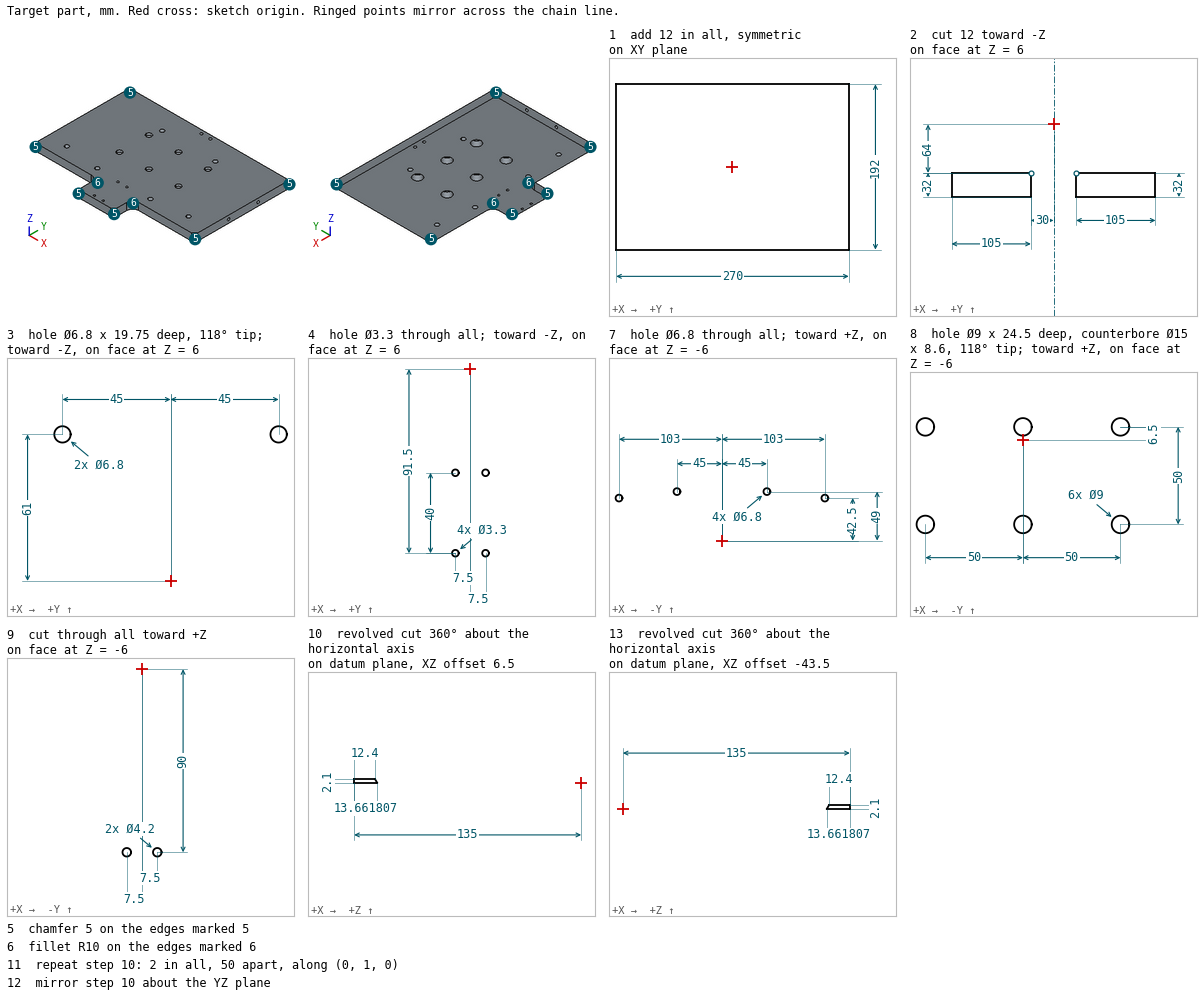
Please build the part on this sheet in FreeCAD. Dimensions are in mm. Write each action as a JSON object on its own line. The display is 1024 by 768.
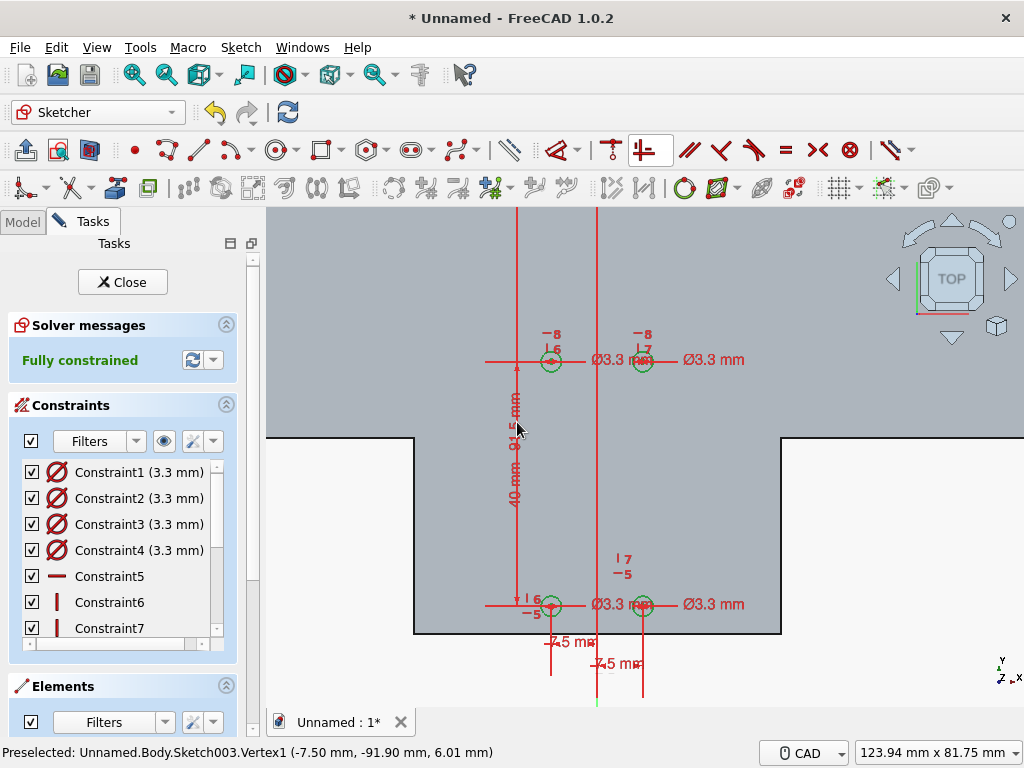
{"action": "left_click", "coordinate": [123, 282]}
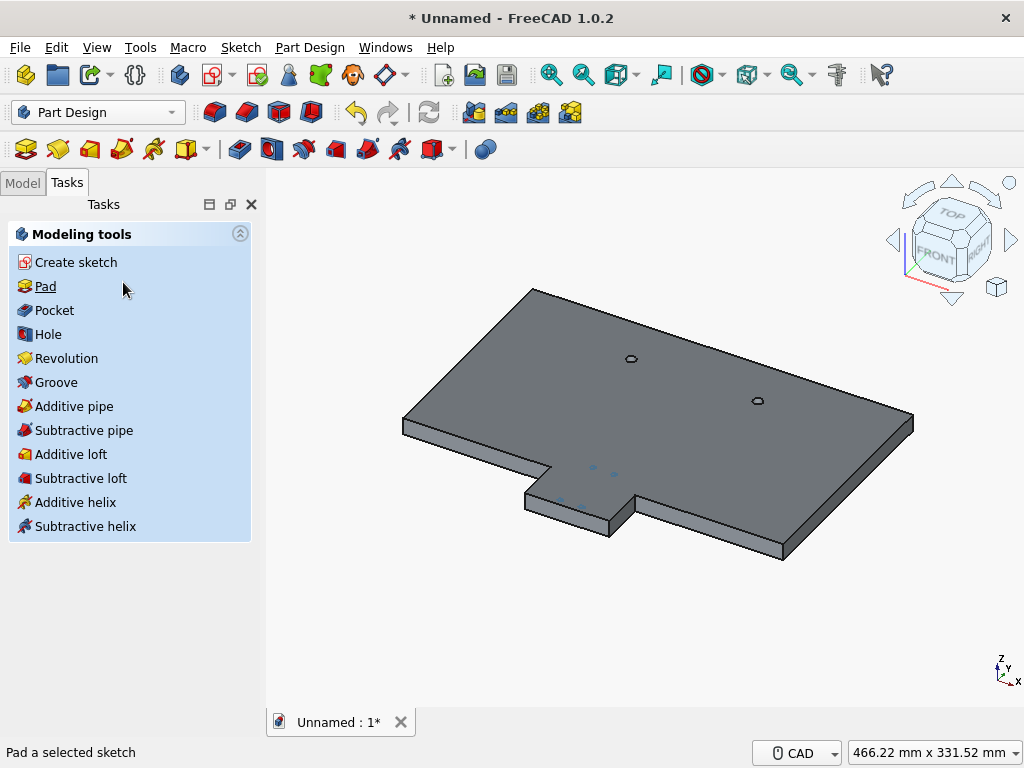
{"action": "left_click", "coordinate": [272, 150]}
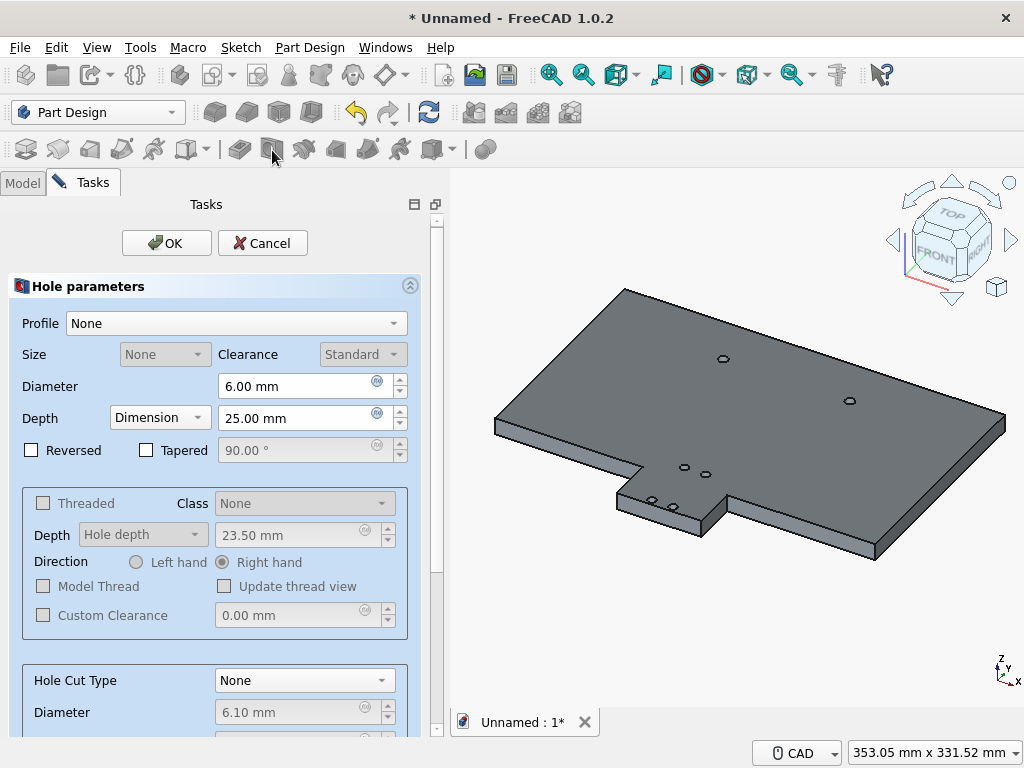
{"action": "triple_click", "coordinate": [305, 386]}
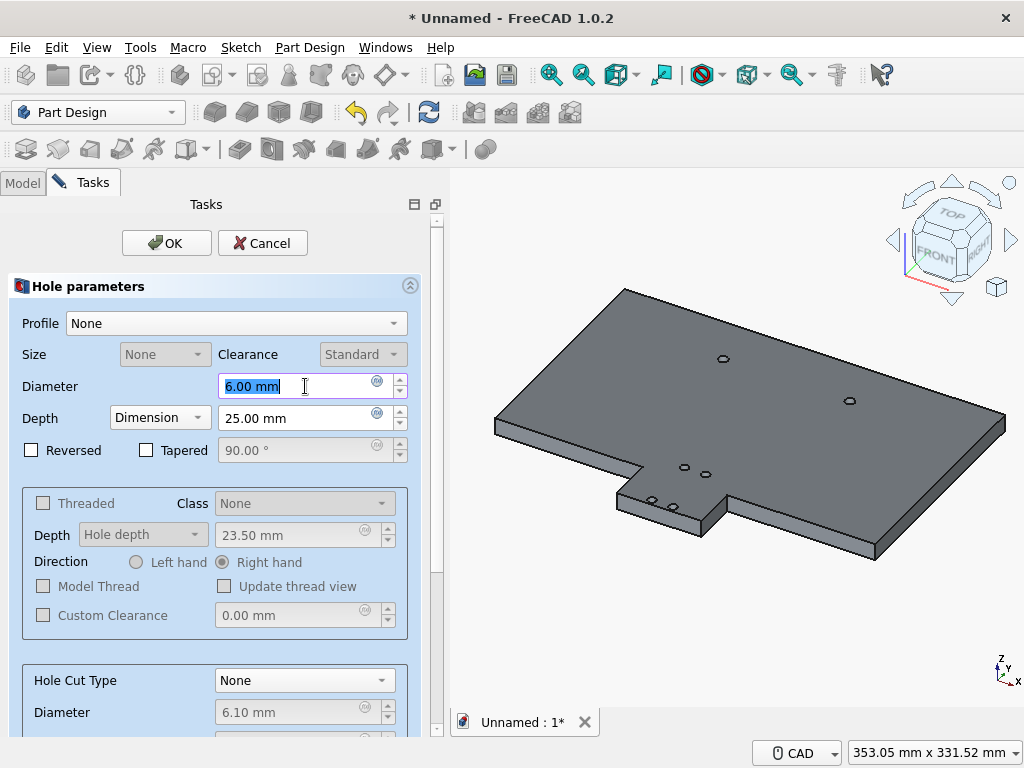
{"action": "type", "text": "3.3"}
{"action": "key", "text": "Tab"}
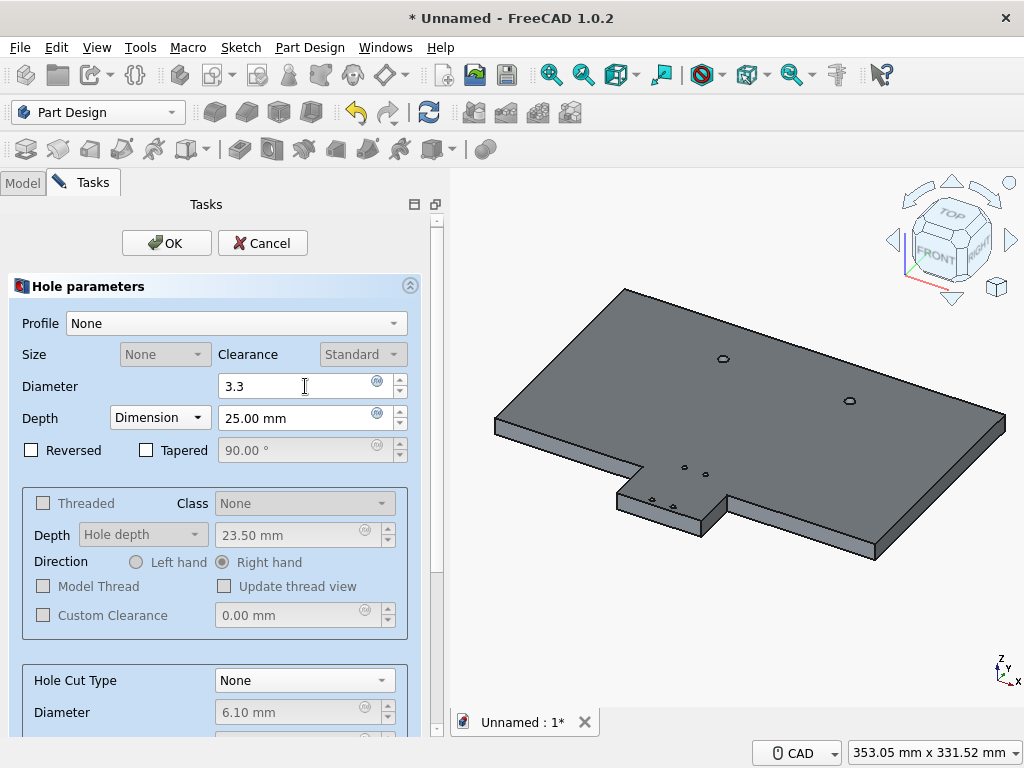
{"action": "left_click", "coordinate": [161, 418]}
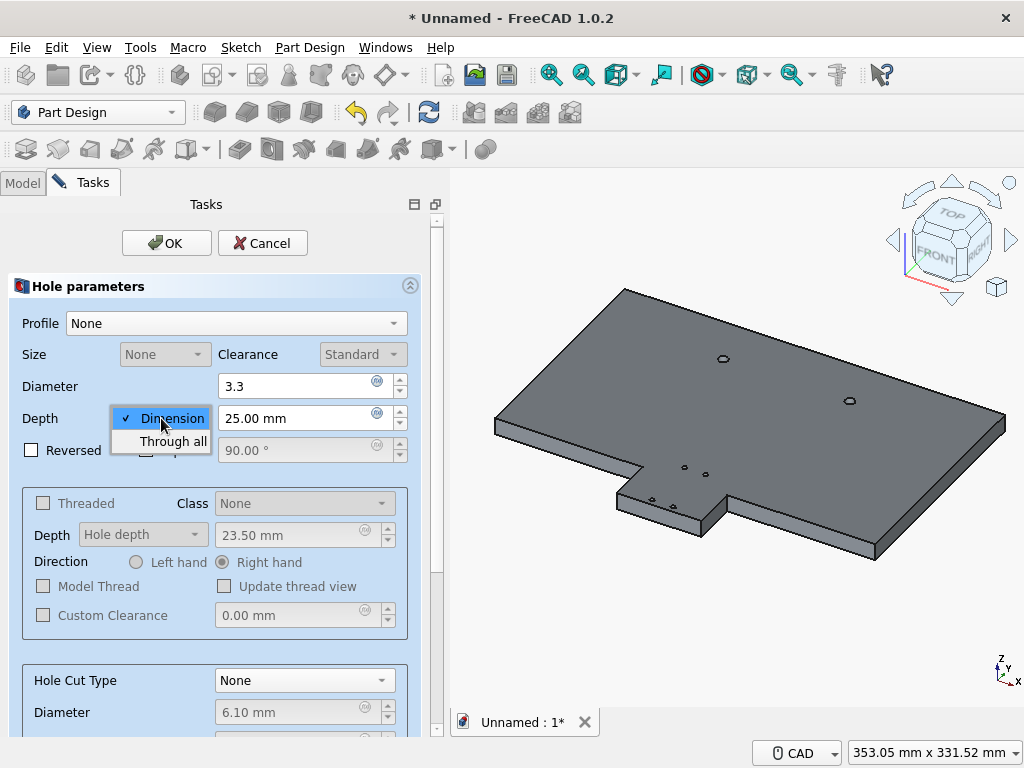
{"action": "left_click", "coordinate": [160, 442]}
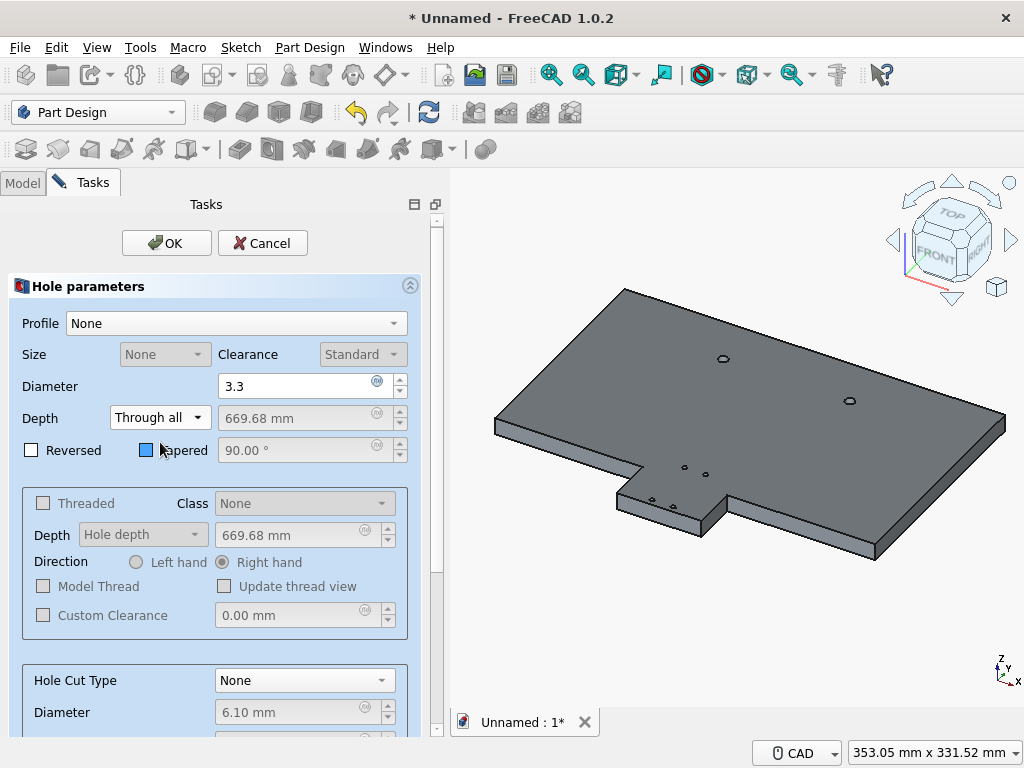
{"action": "left_click", "coordinate": [167, 243]}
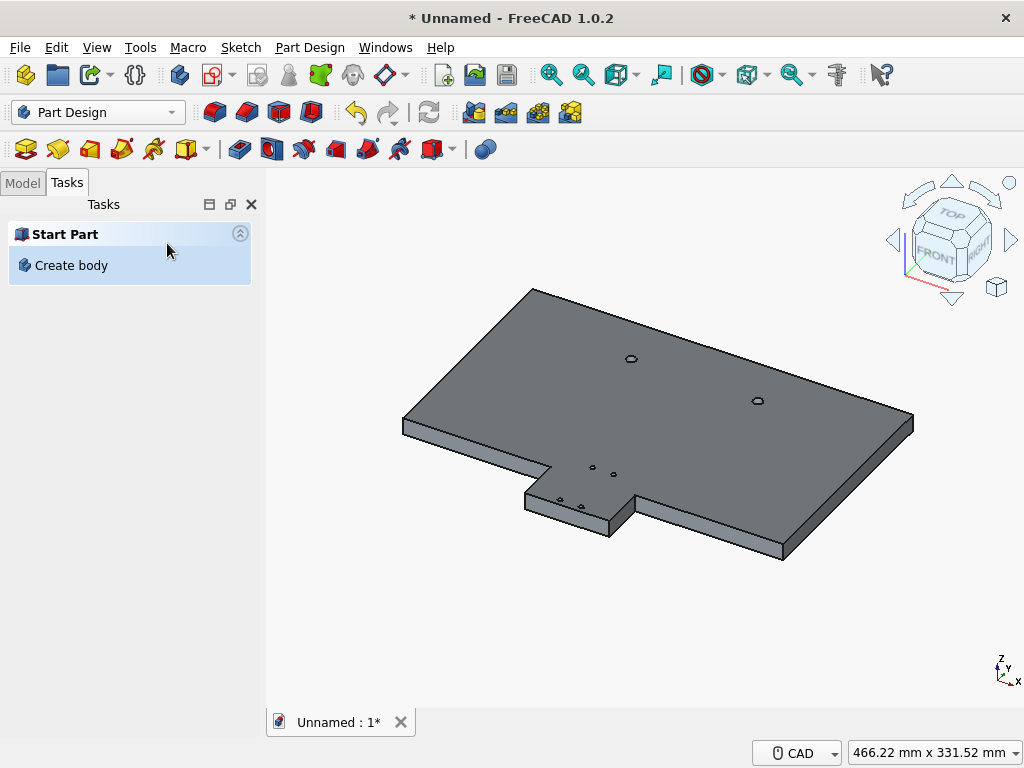
{"action": "left_click", "coordinate": [609, 528]}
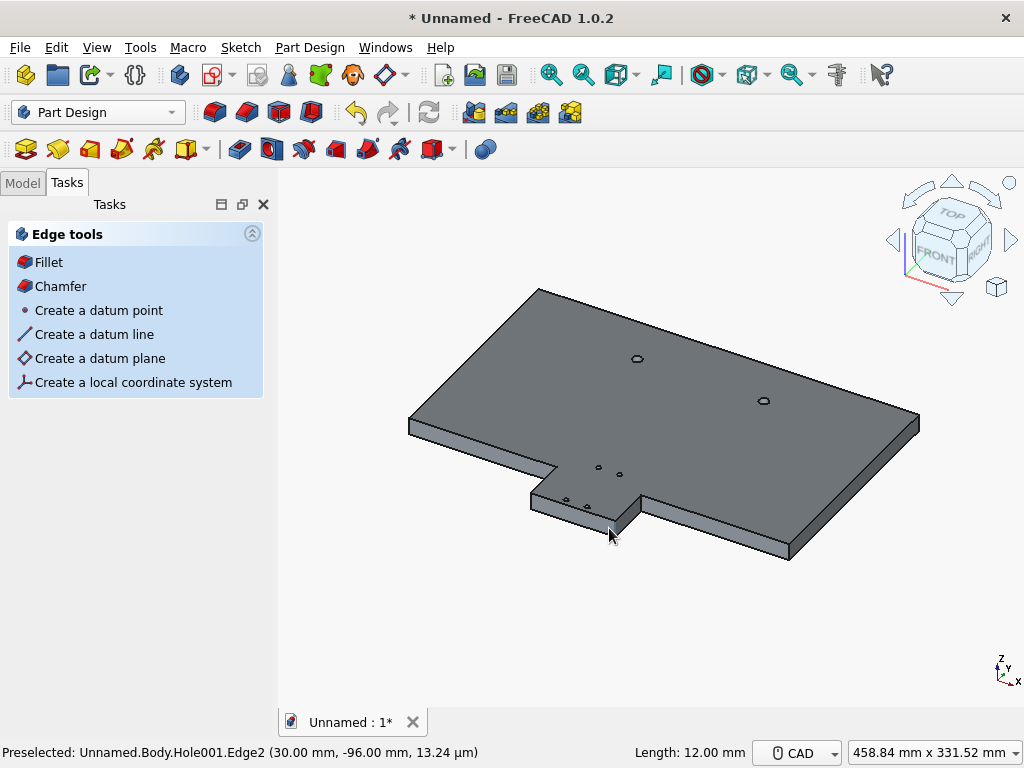
{"action": "left_click", "coordinate": [789, 551], "text": "ctrl"}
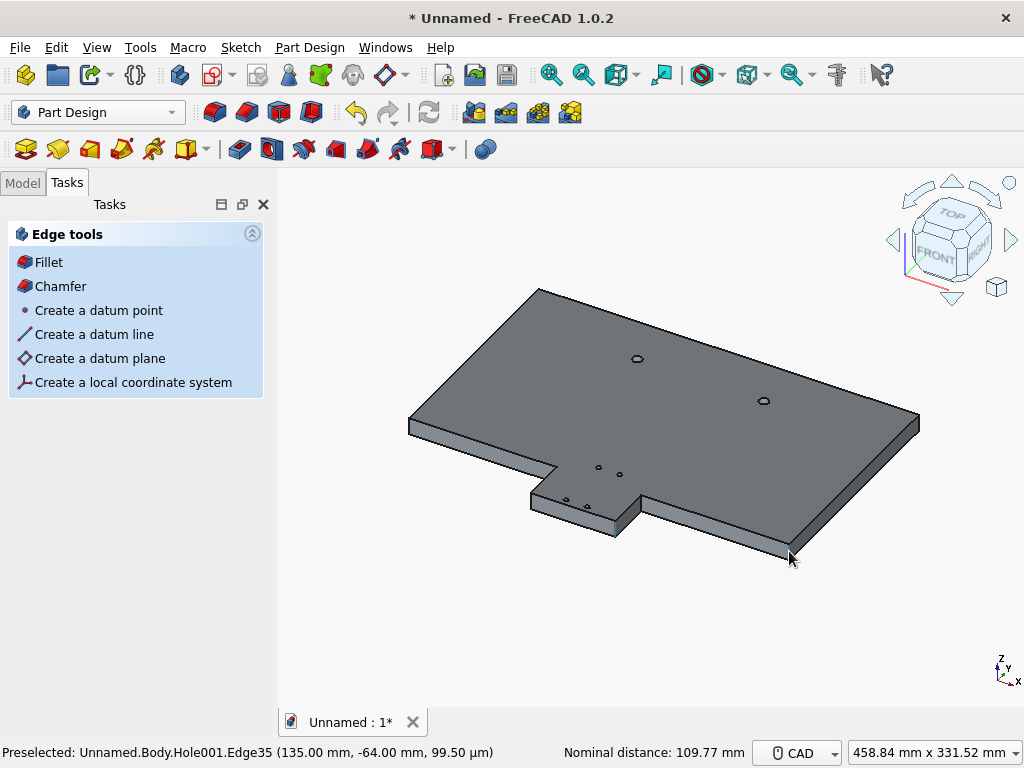
{"action": "scroll", "coordinate": [409, 425], "scroll_direction": "up", "scroll_amount": 4}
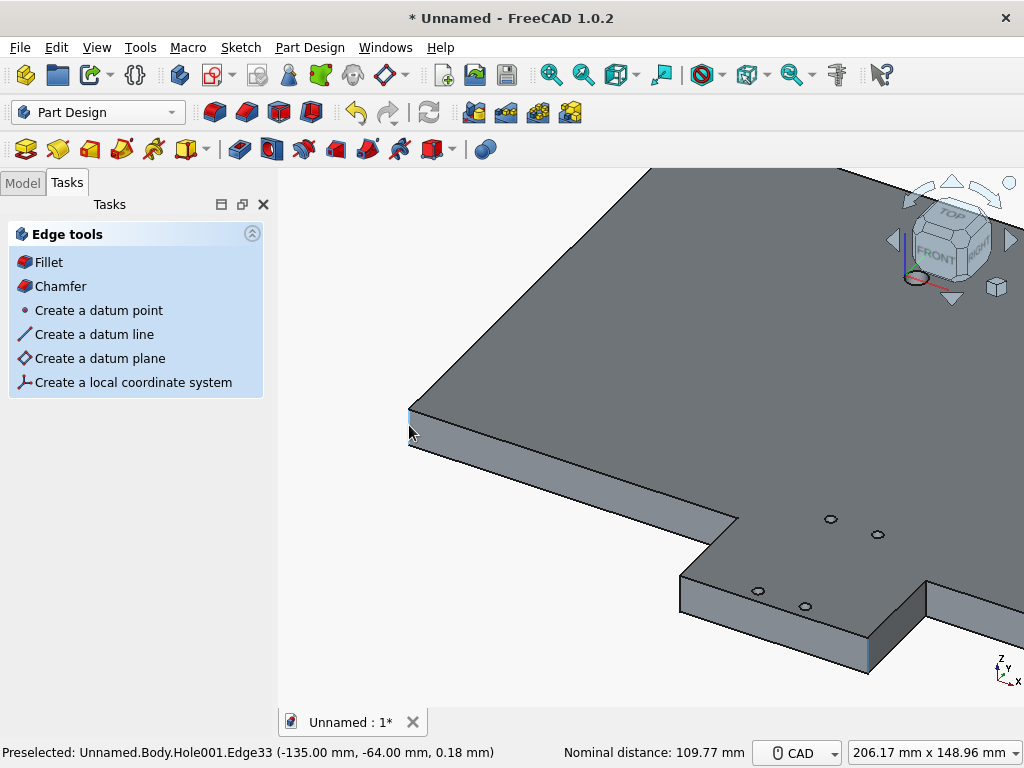
{"action": "key", "text": "v f"}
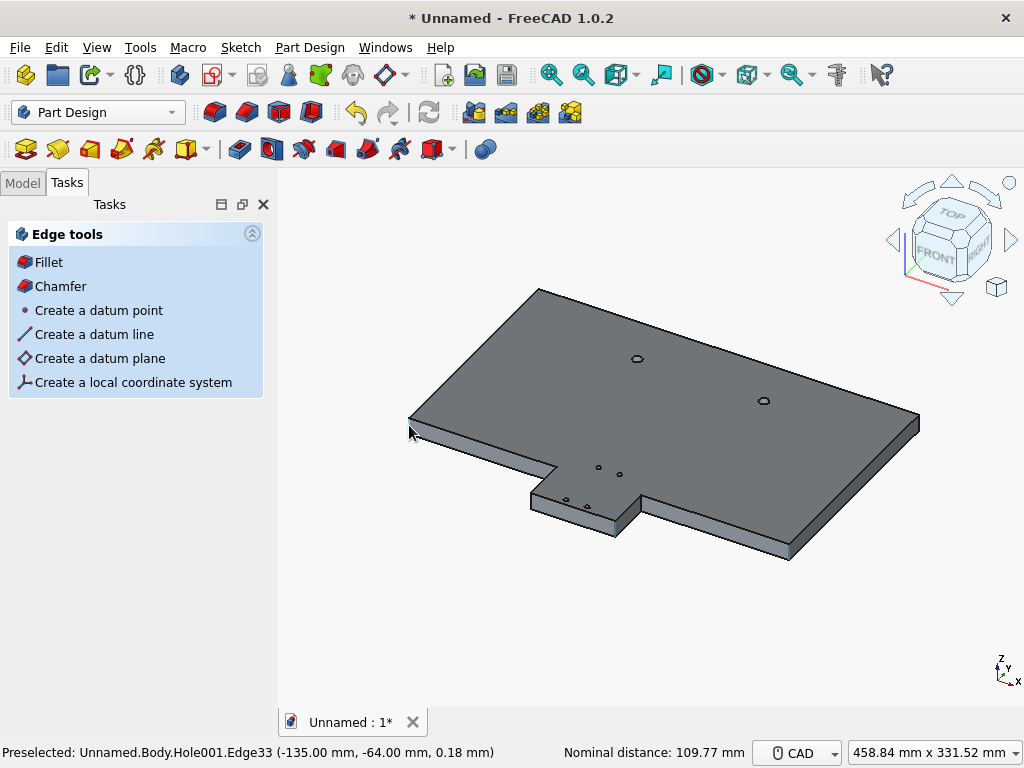
{"action": "key", "text": "0"}